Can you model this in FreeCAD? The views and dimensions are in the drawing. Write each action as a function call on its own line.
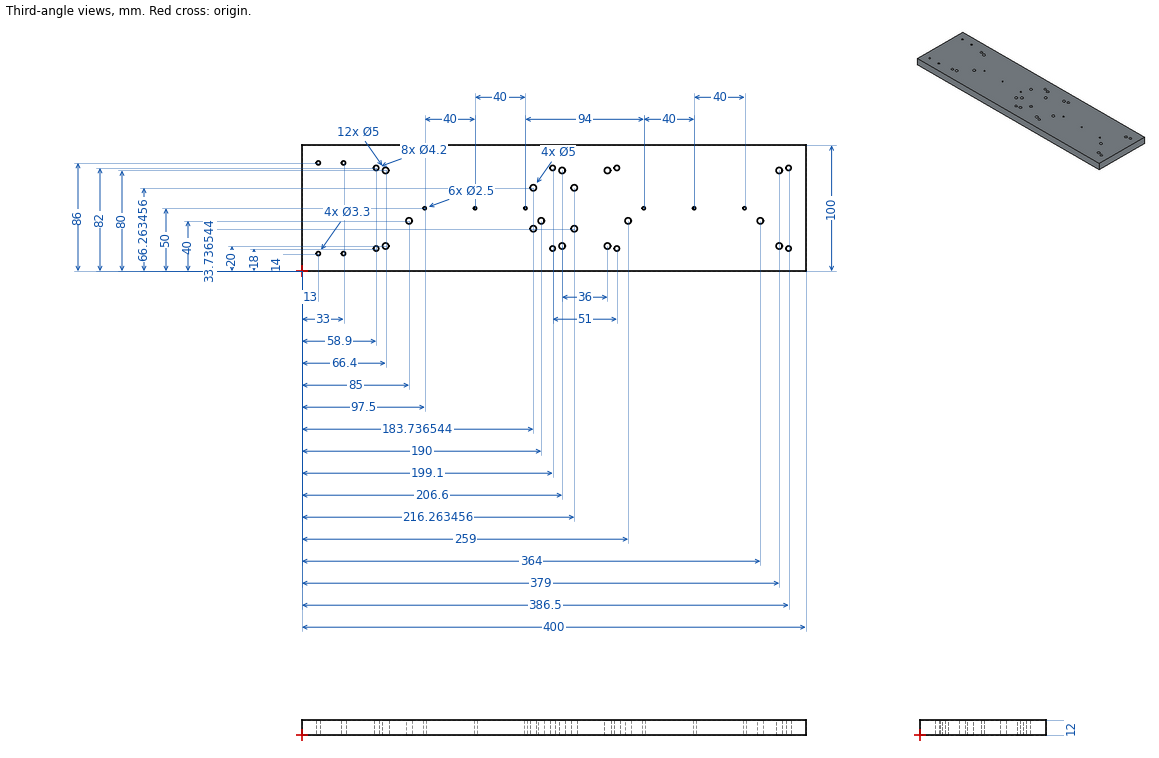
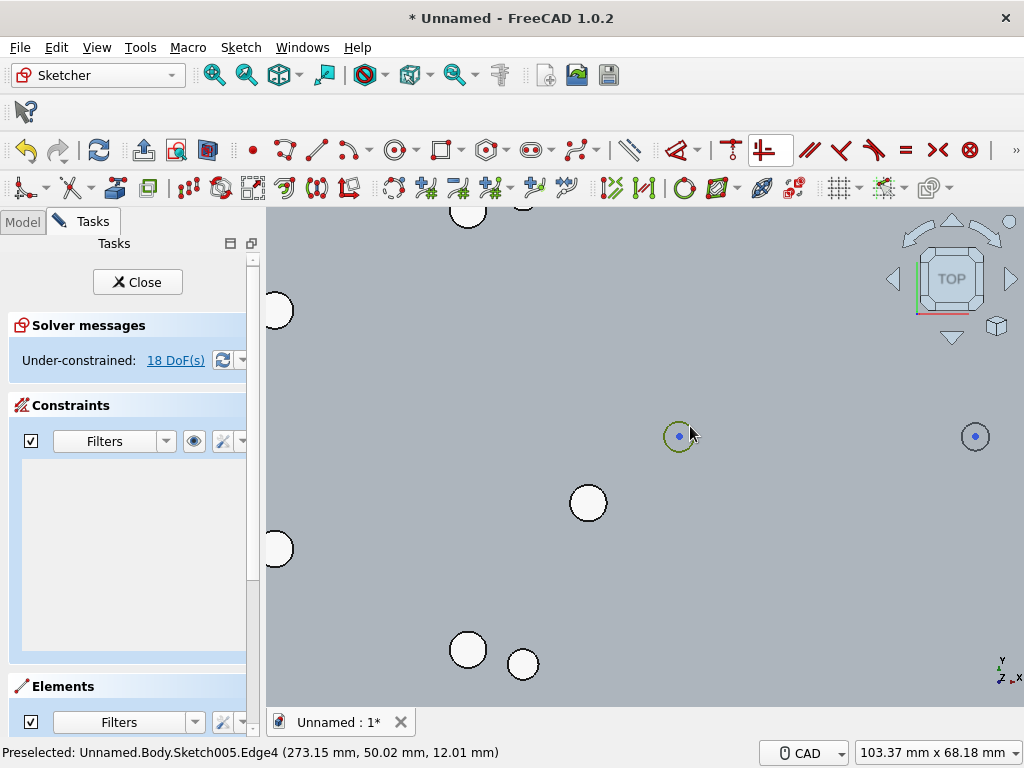
scroll(694, 427, down, 9)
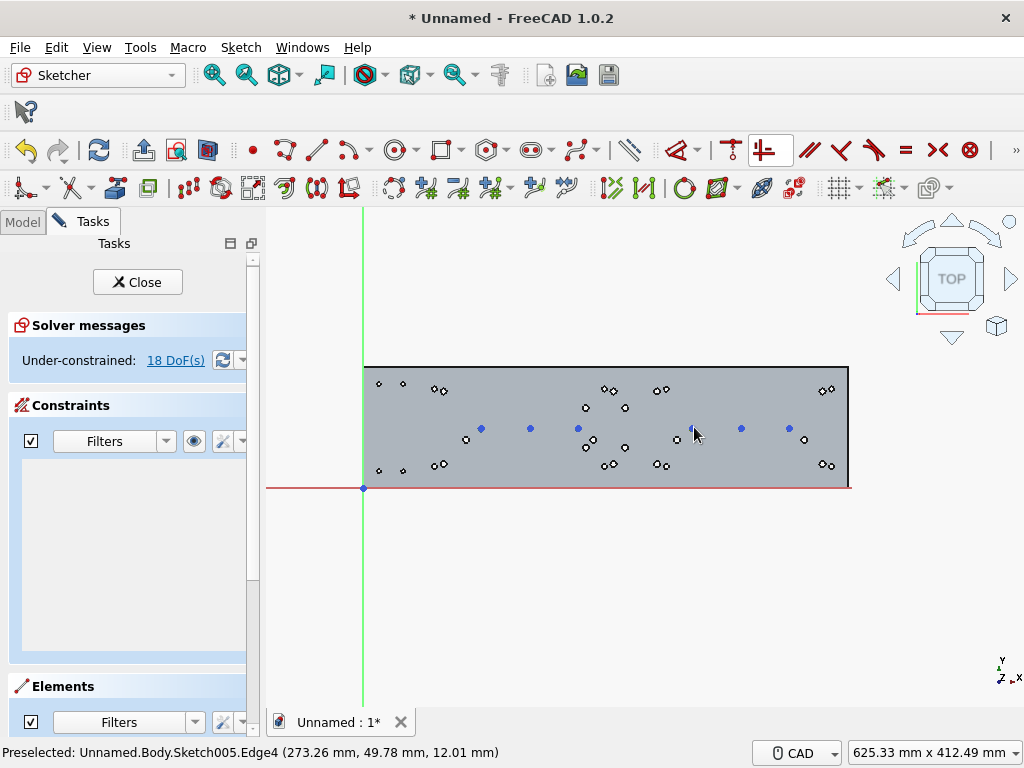
scroll(743, 427, up, 10)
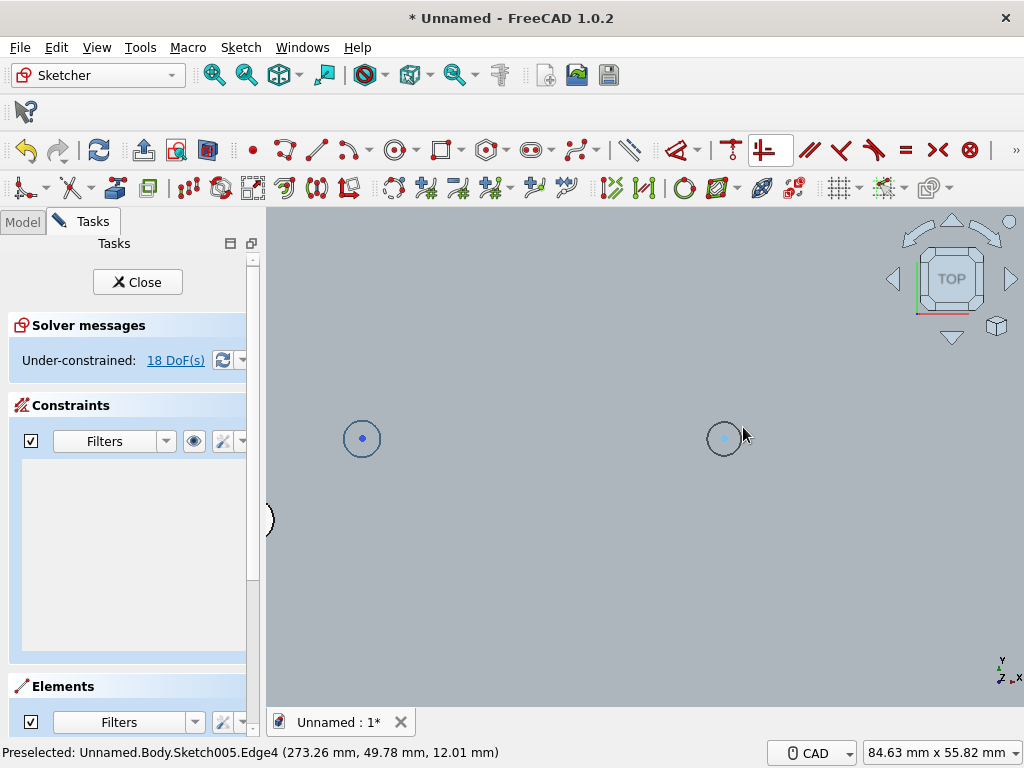
click(736, 427)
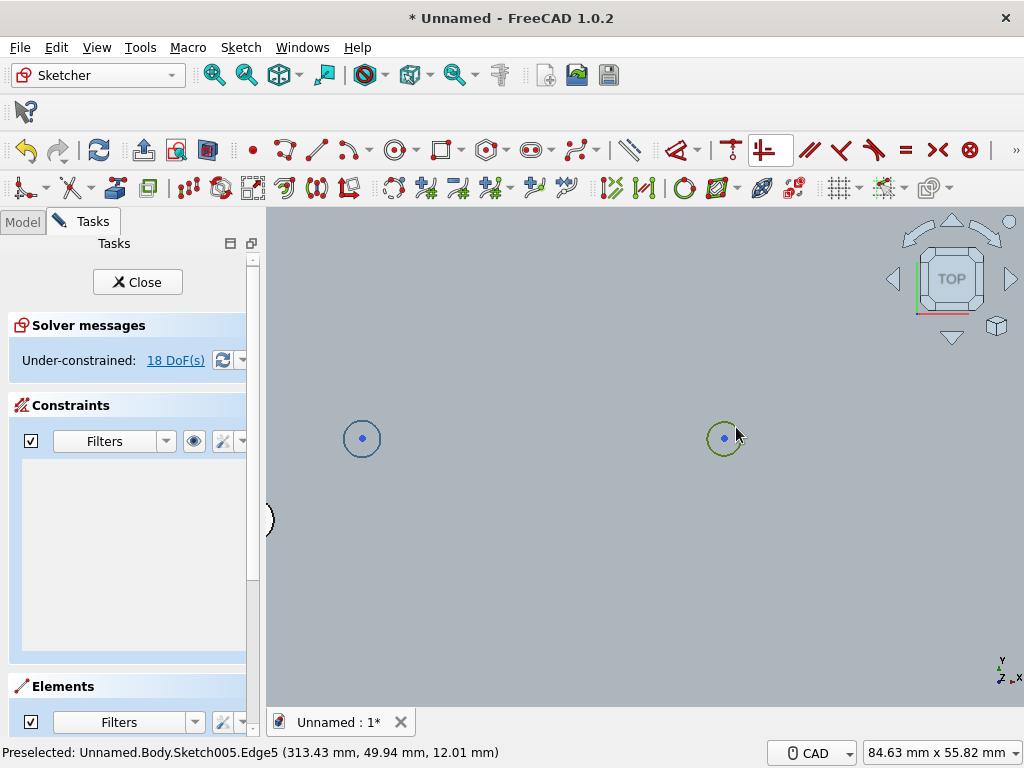
scroll(743, 427, down, 10)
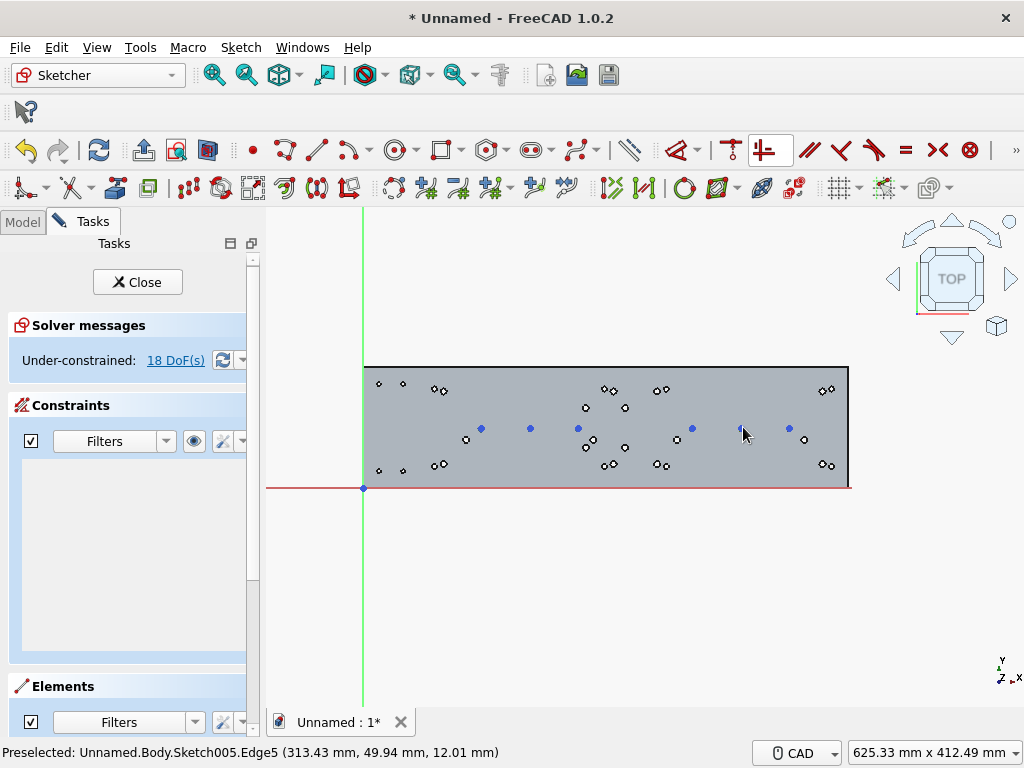
scroll(791, 427, up, 9)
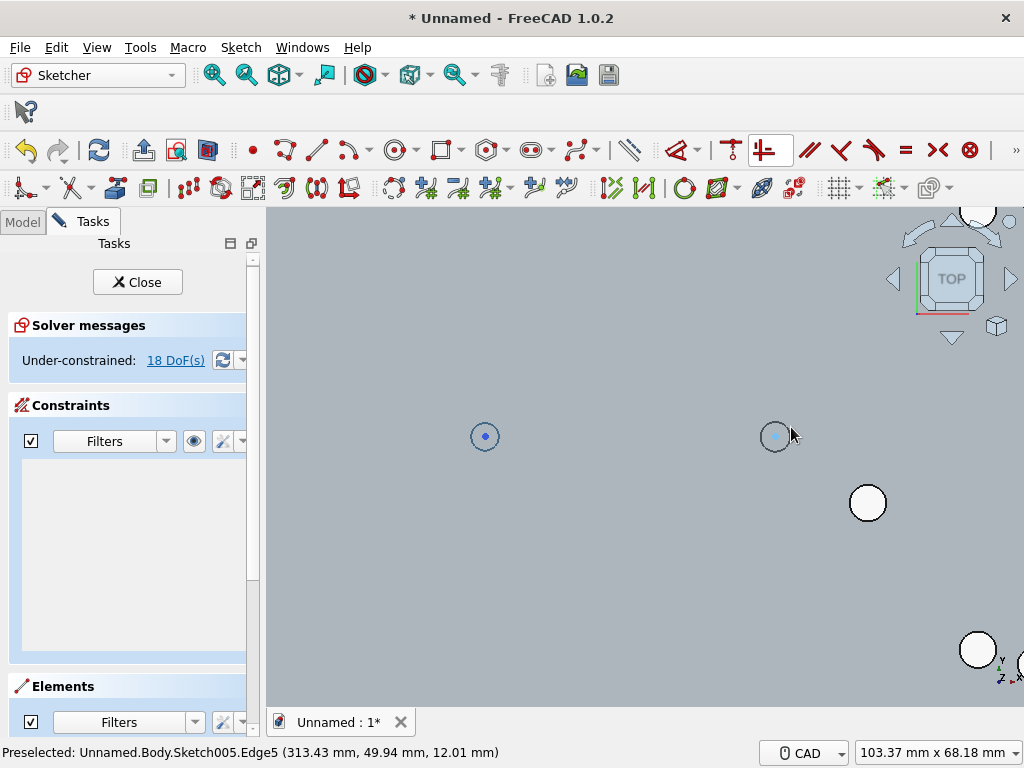
click(786, 426)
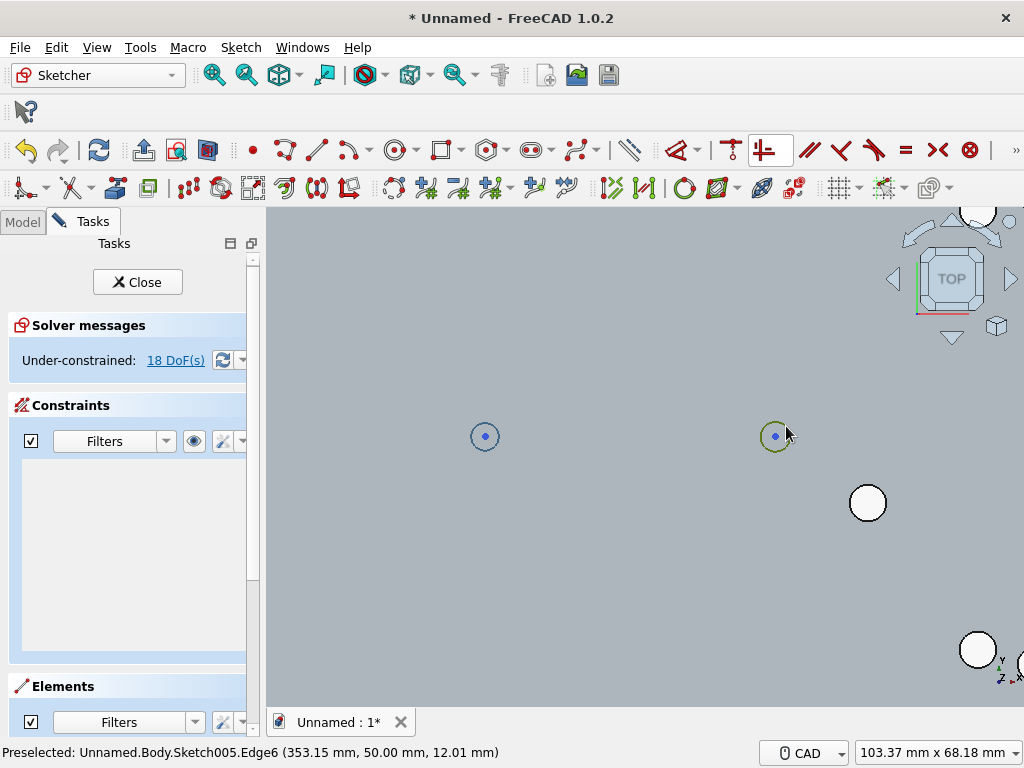
click(906, 150)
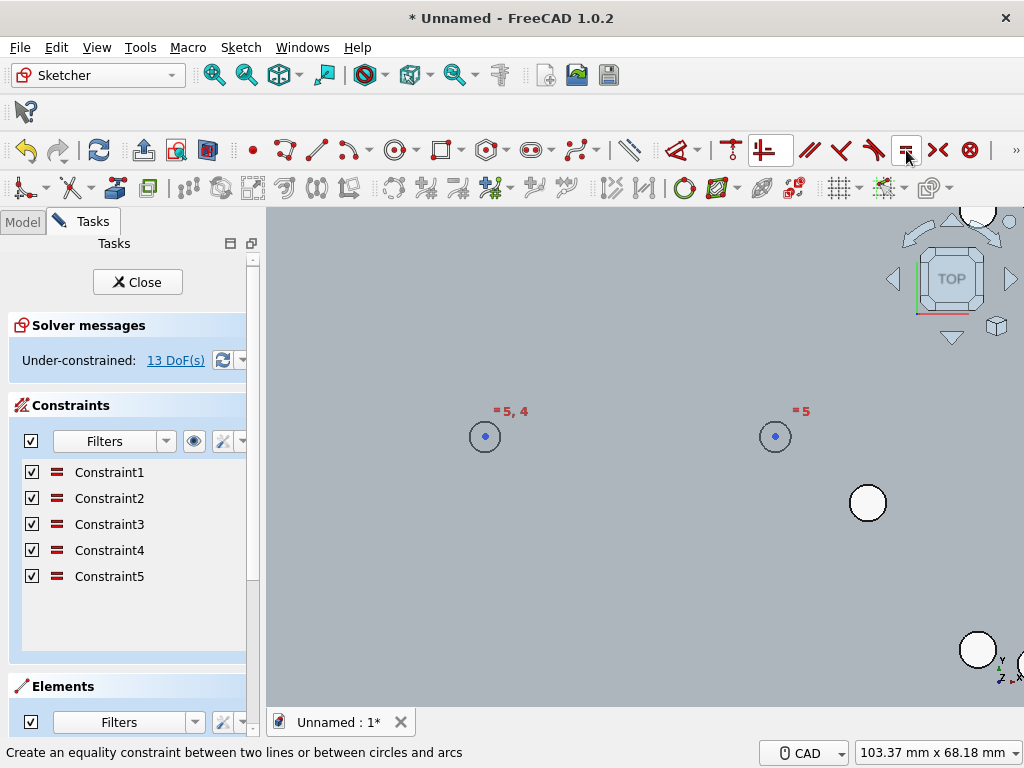
scroll(791, 427, down, 9)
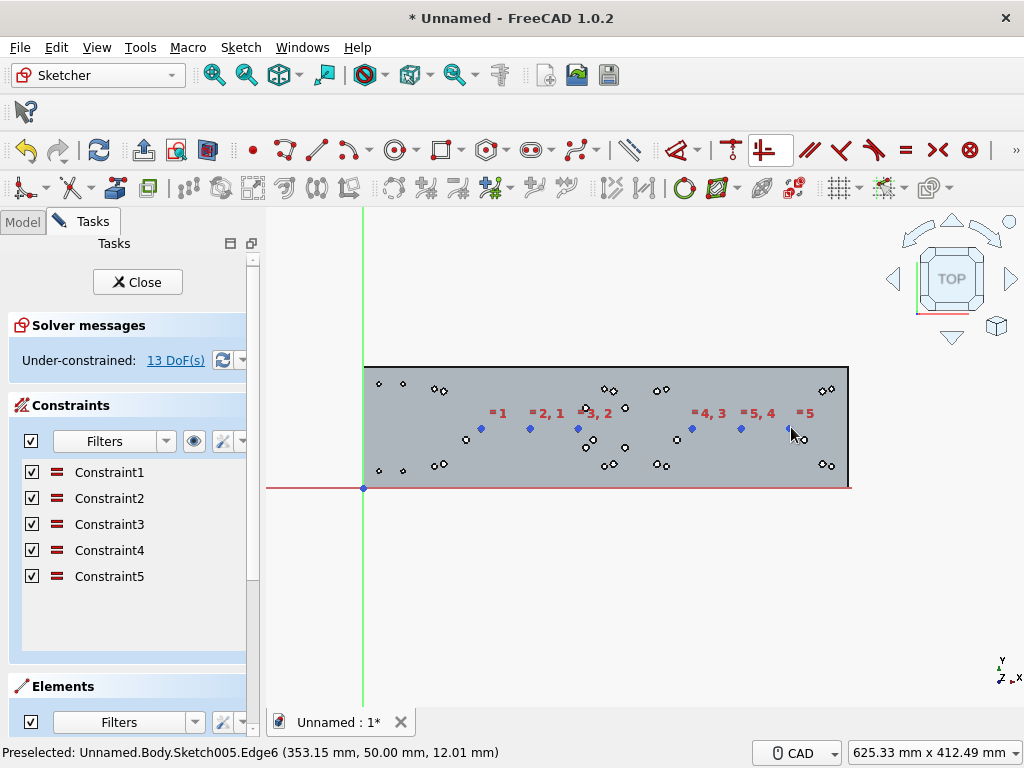
click(481, 429)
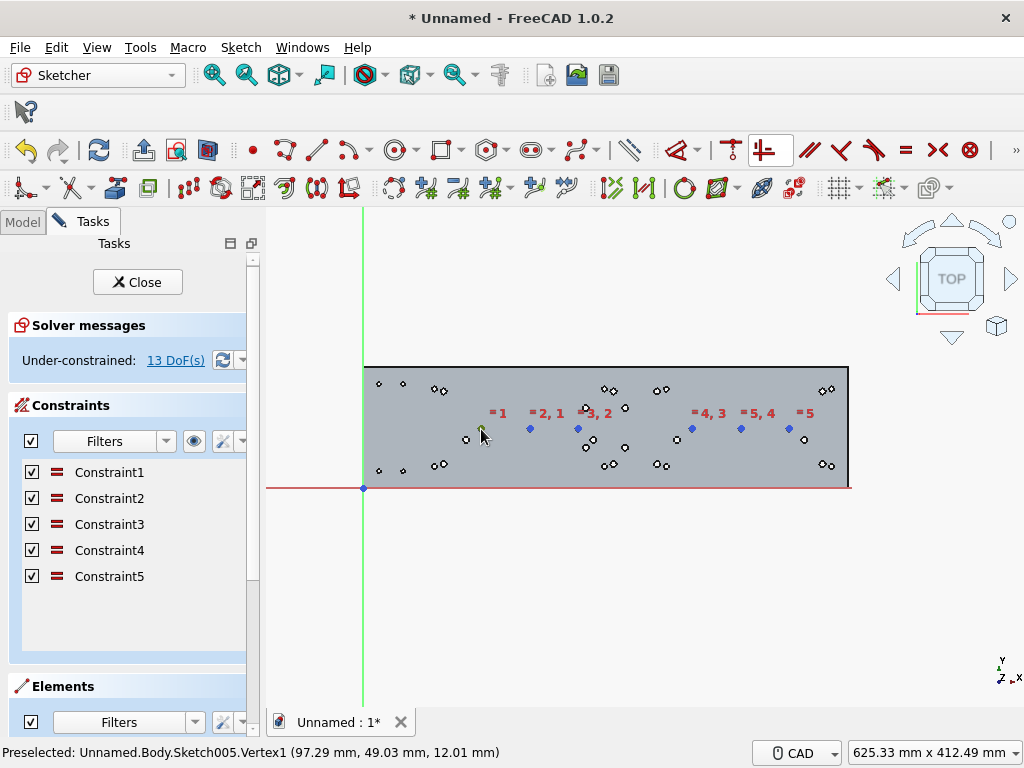
click(530, 429)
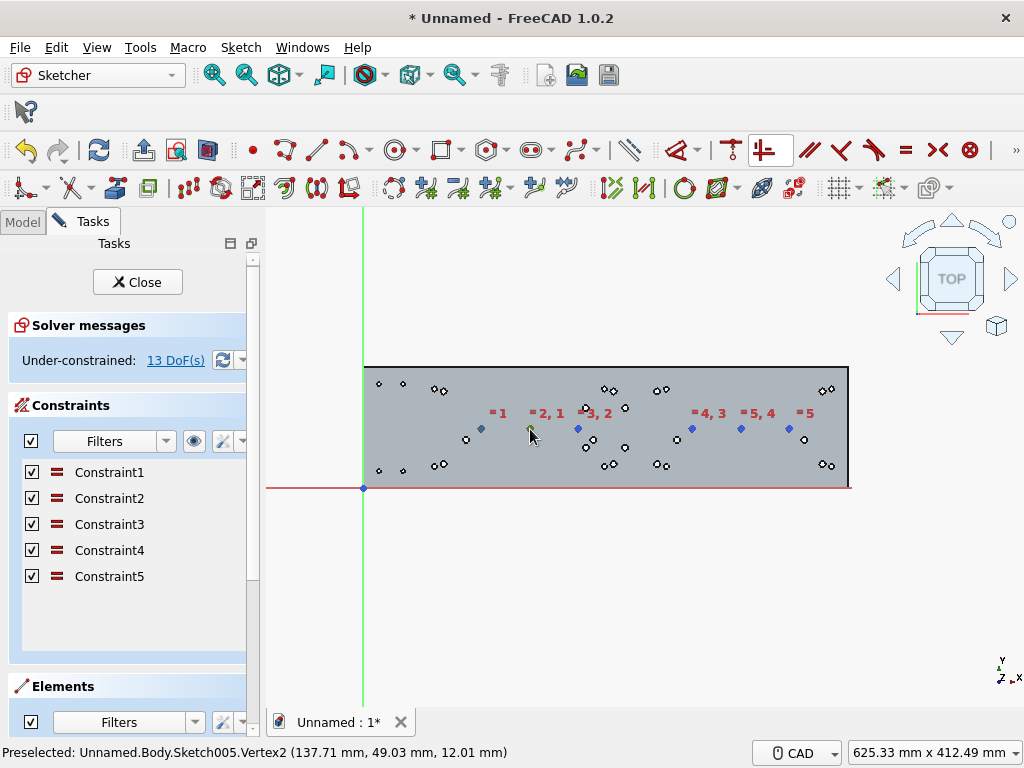
click(788, 150)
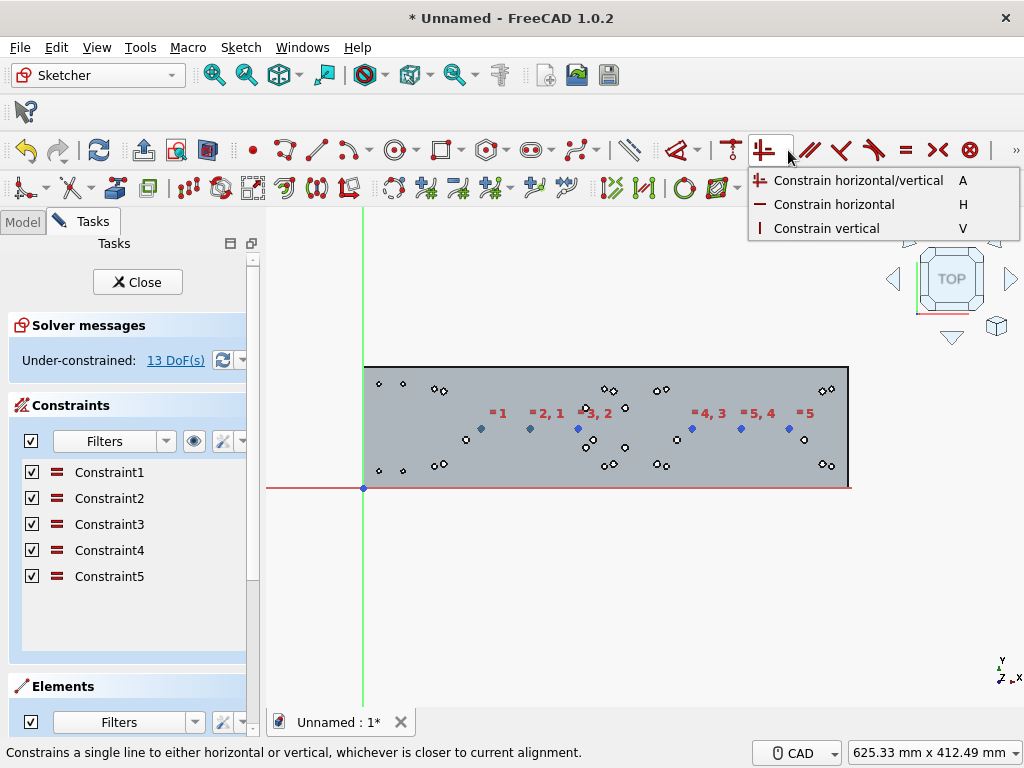
click(884, 204)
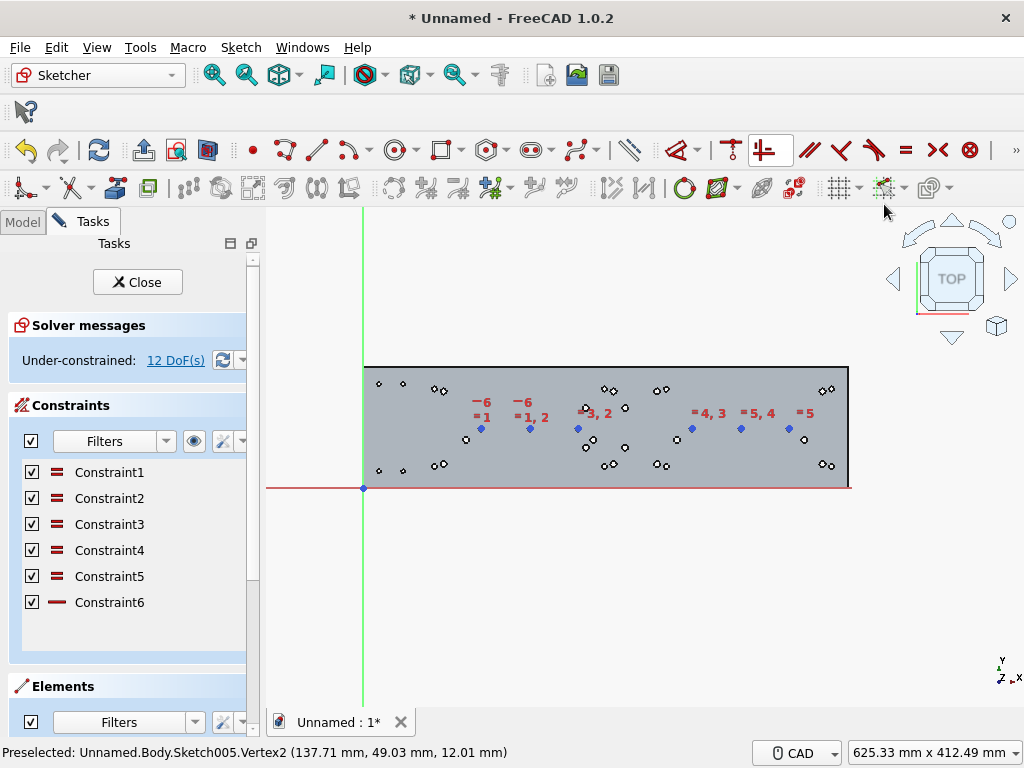
click(530, 429)